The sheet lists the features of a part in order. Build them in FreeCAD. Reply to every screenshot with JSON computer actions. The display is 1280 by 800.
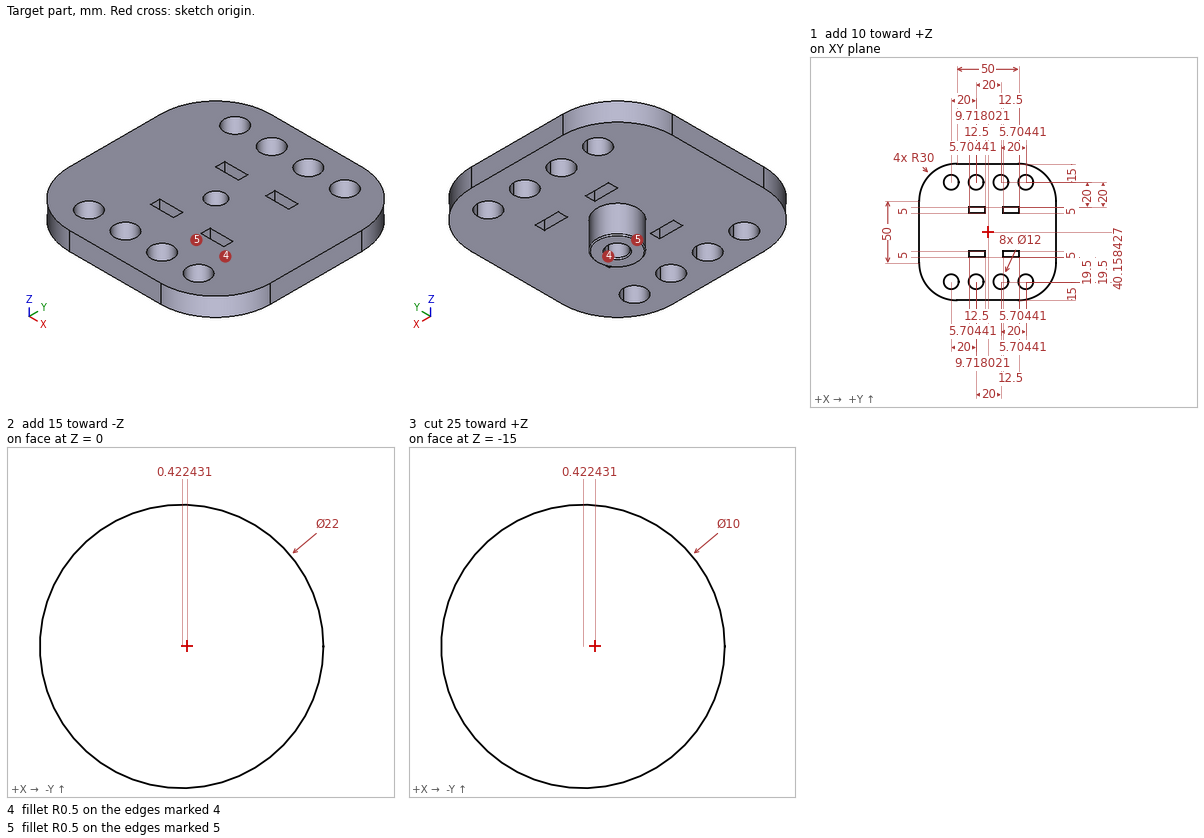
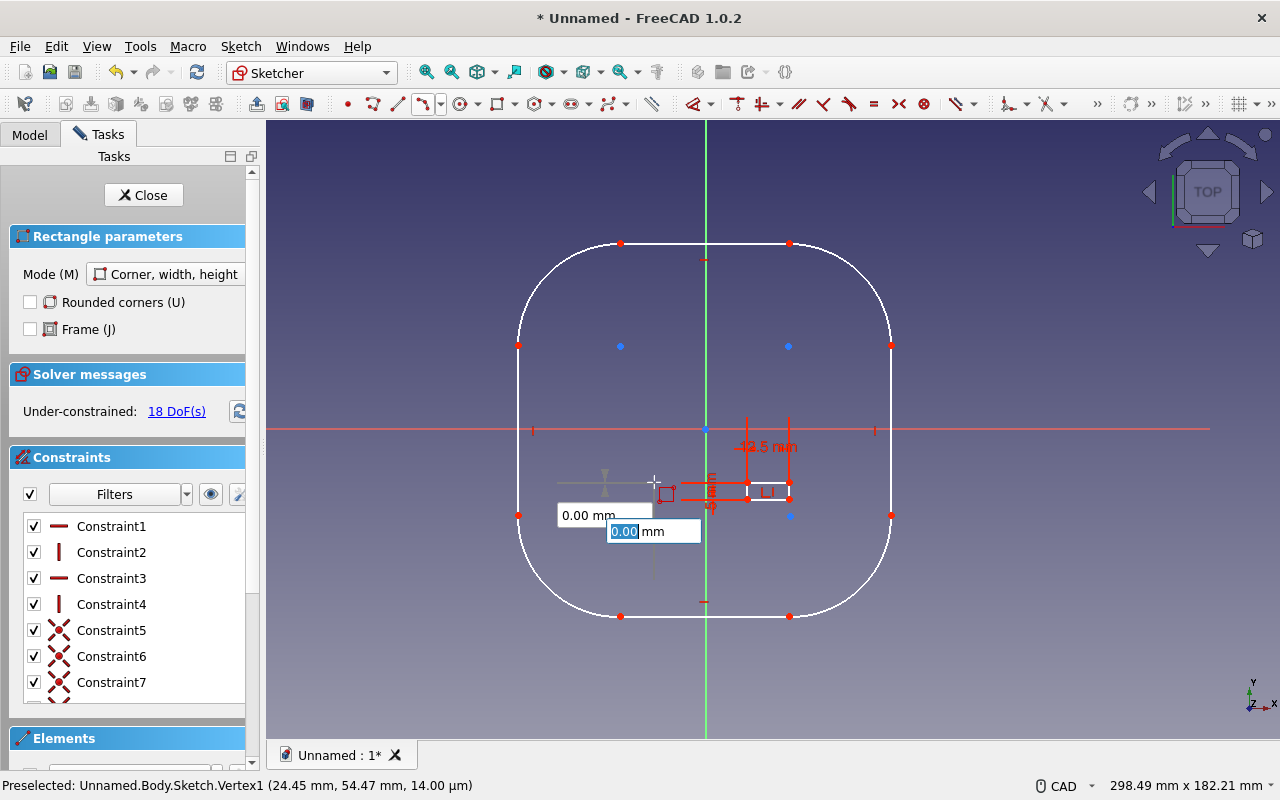
{"action": "scroll", "coordinate": [696, 499], "scroll_direction": "up", "scroll_amount": 3}
{"action": "mouse_move", "coordinate": [696, 499]}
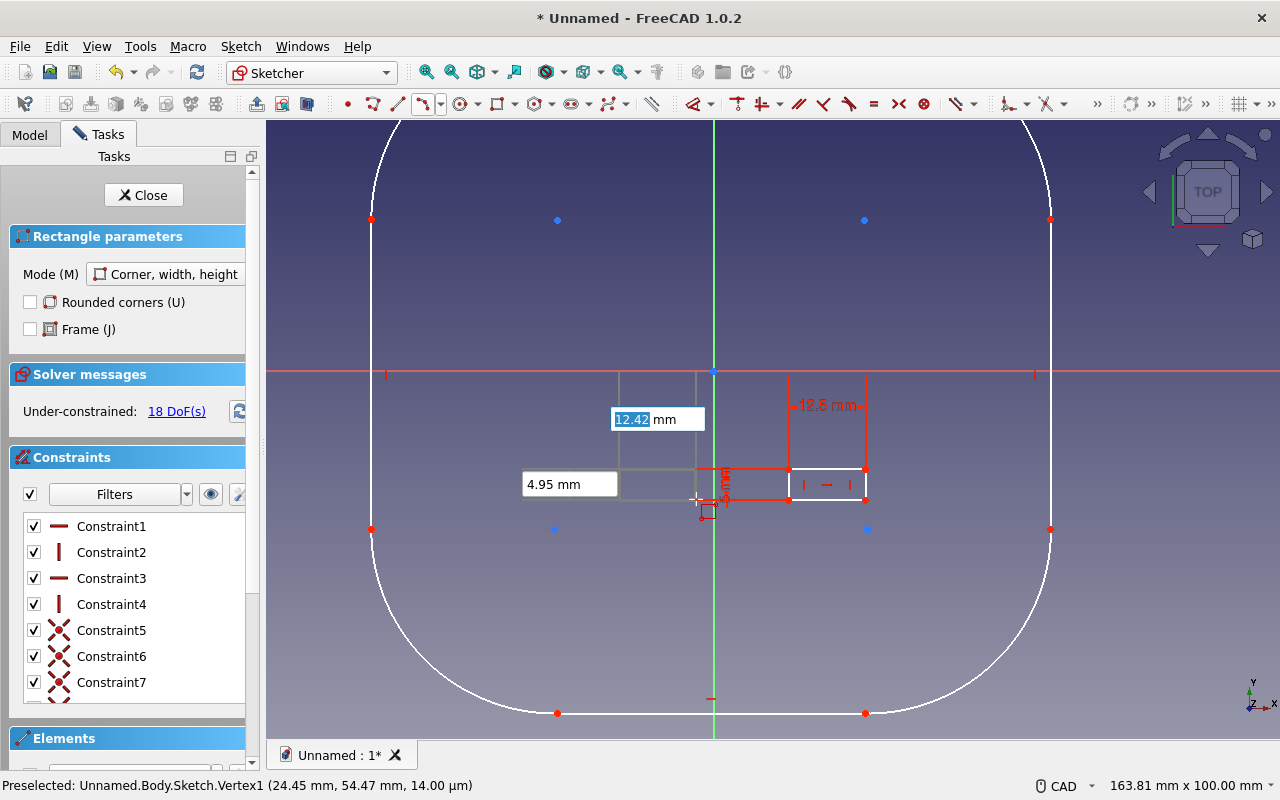
{"action": "type", "text": "12.5"}
{"action": "key", "text": "Tab"}
{"action": "type", "text": "5"}
{"action": "key", "text": "Return"}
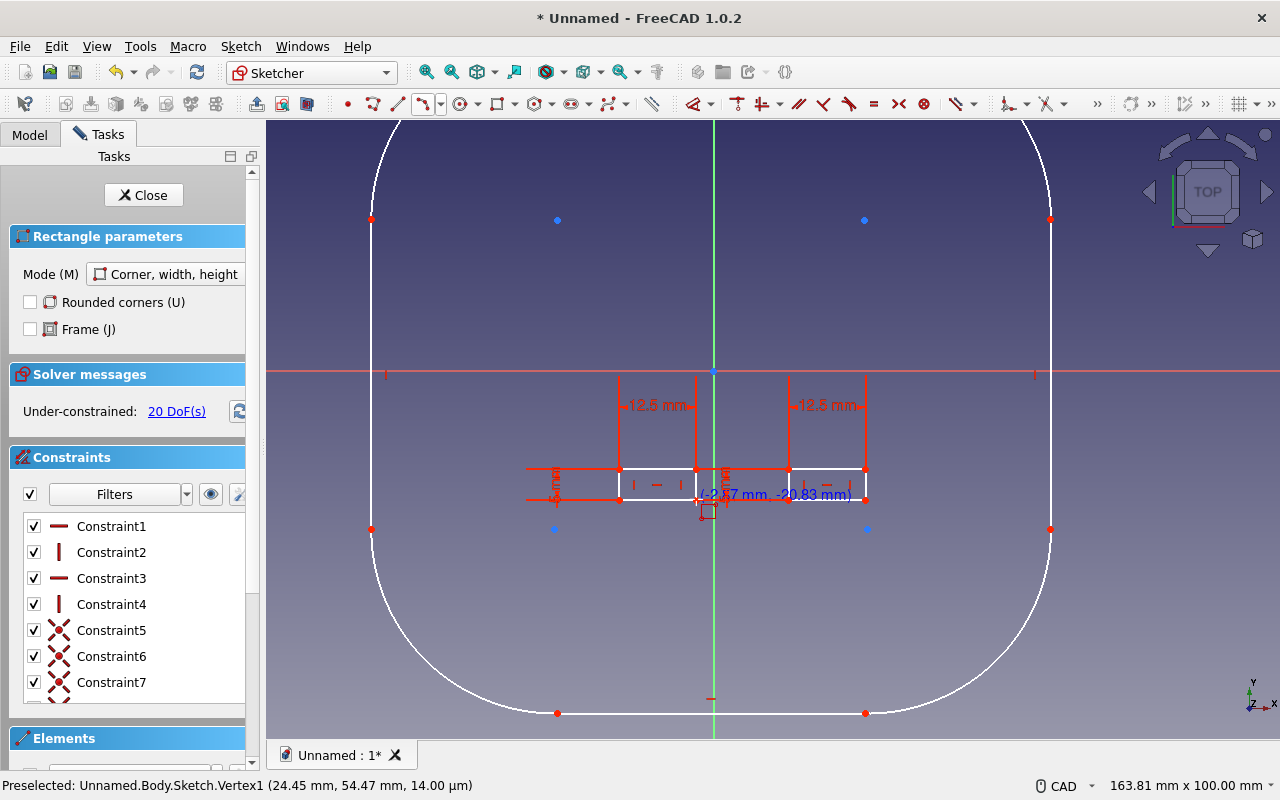
{"action": "left_click", "coordinate": [789, 248]}
{"action": "mouse_move", "coordinate": [866, 279]}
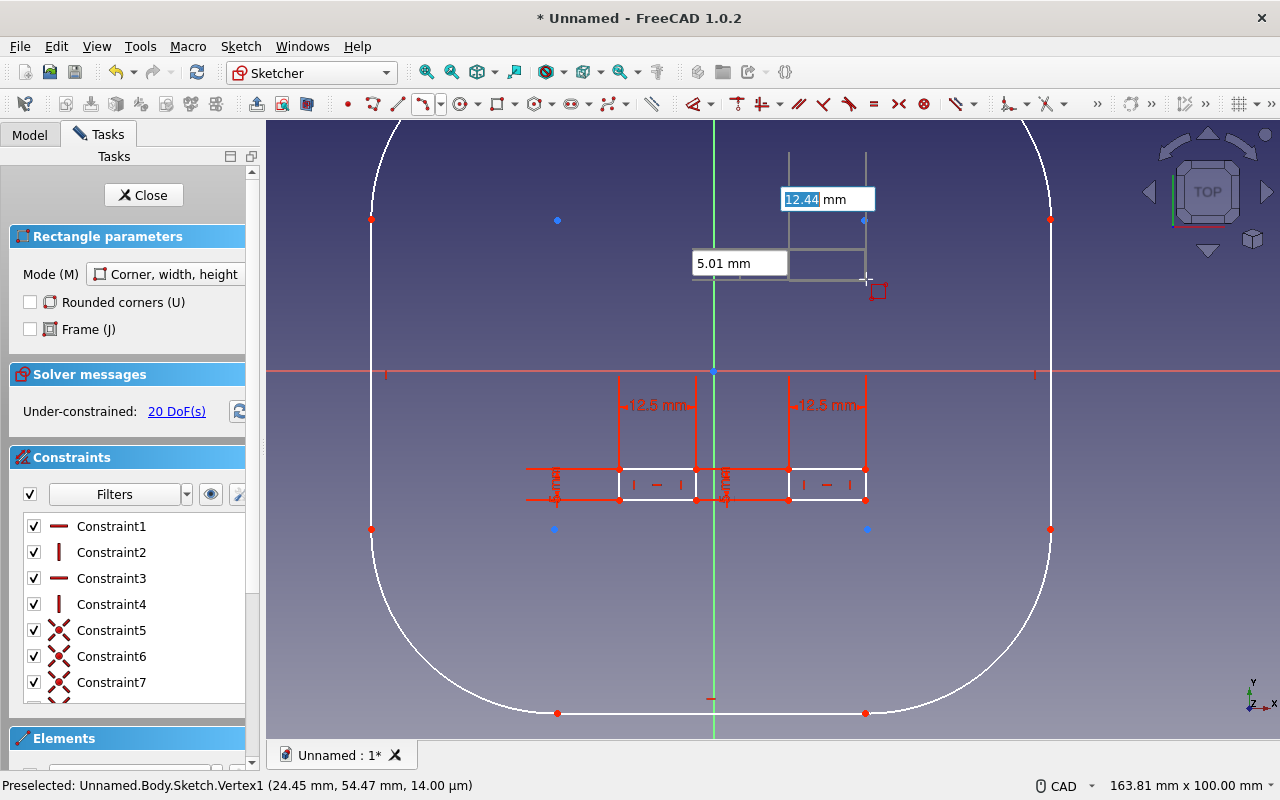
{"action": "type", "text": "12.5"}
{"action": "key", "text": "Tab"}
{"action": "type", "text": "5"}
{"action": "key", "text": "Return"}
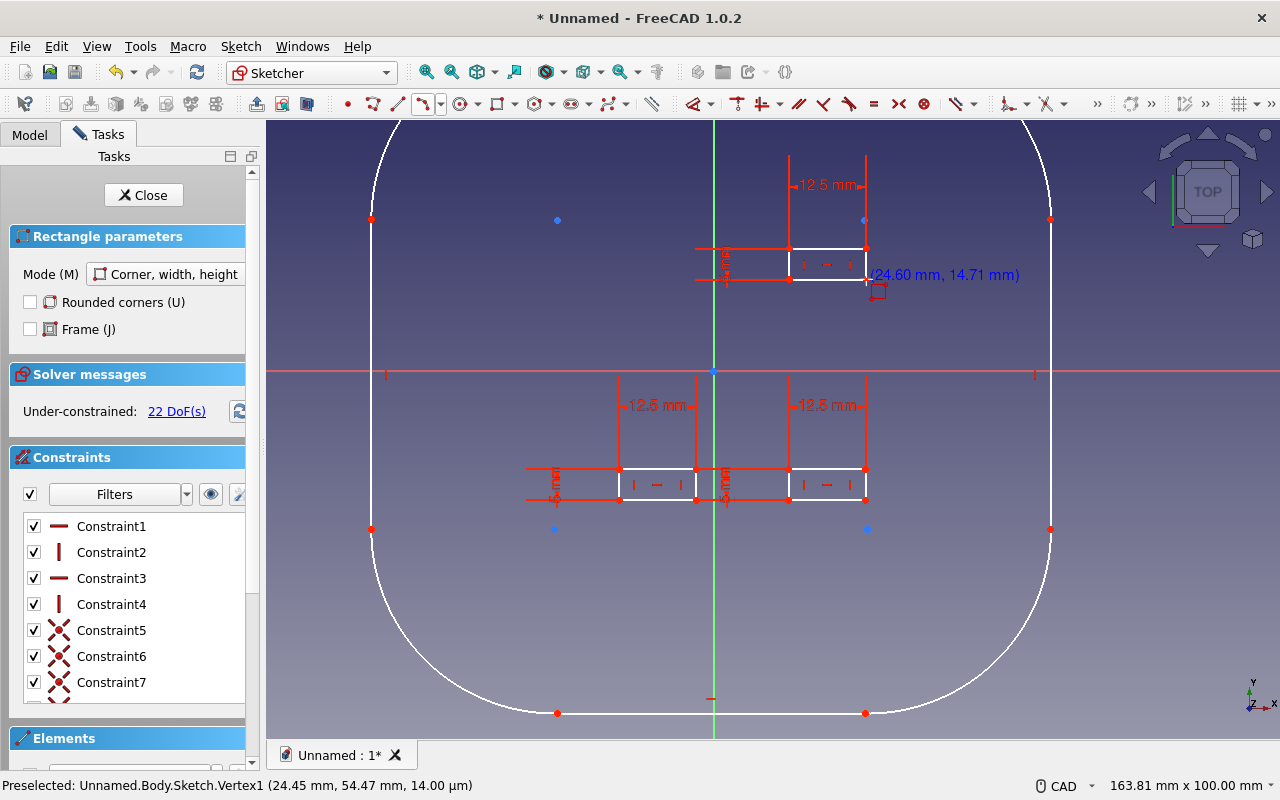
{"action": "left_click", "coordinate": [618, 248]}
{"action": "mouse_move", "coordinate": [696, 279]}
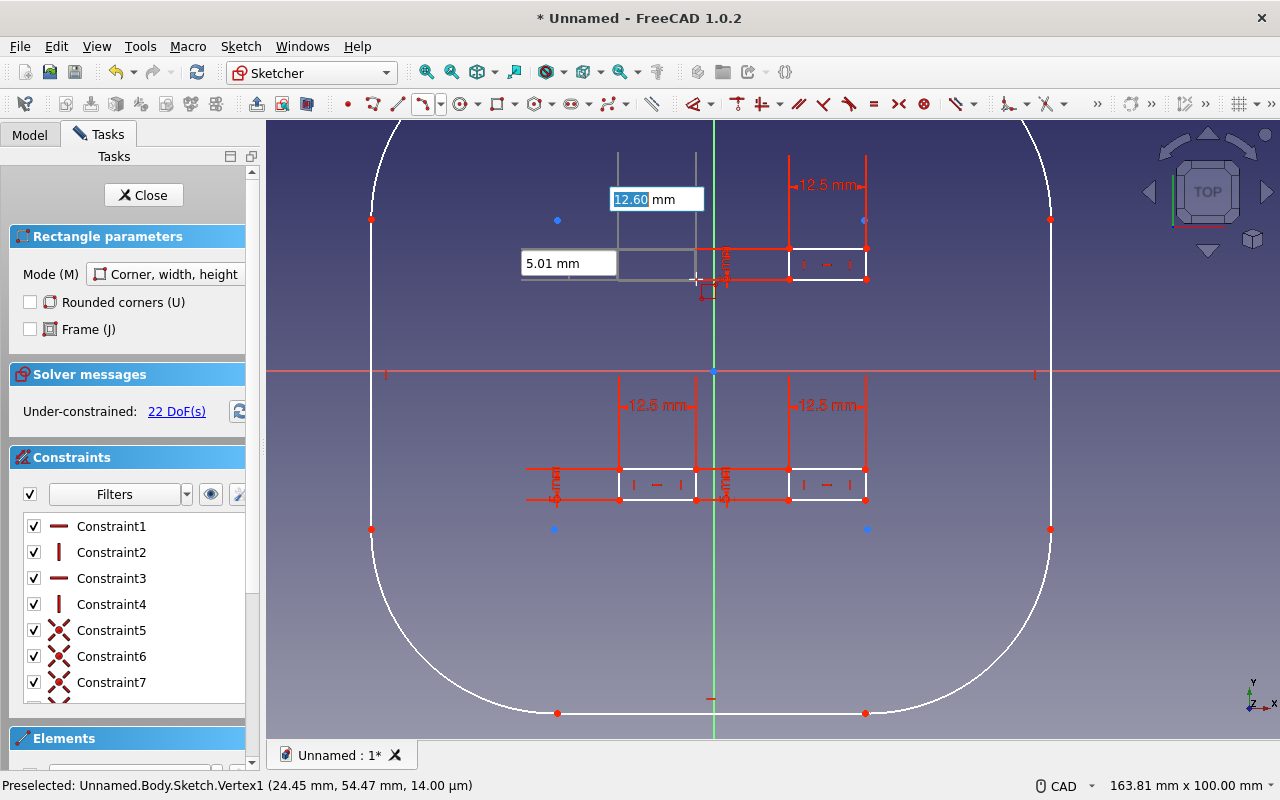
{"action": "type", "text": "12.5"}
{"action": "key", "text": "Tab"}
{"action": "type", "text": "5"}
{"action": "key", "text": "Return"}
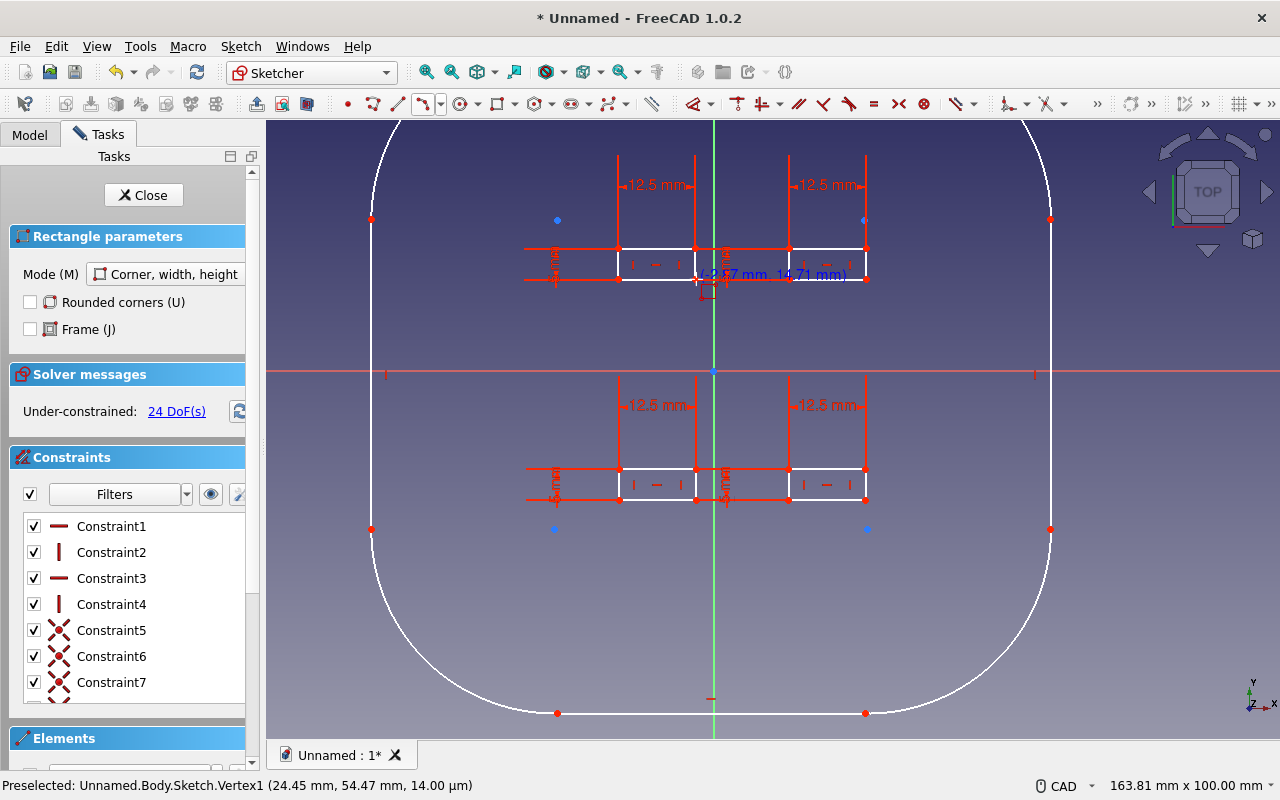
{"action": "key", "text": "g c"}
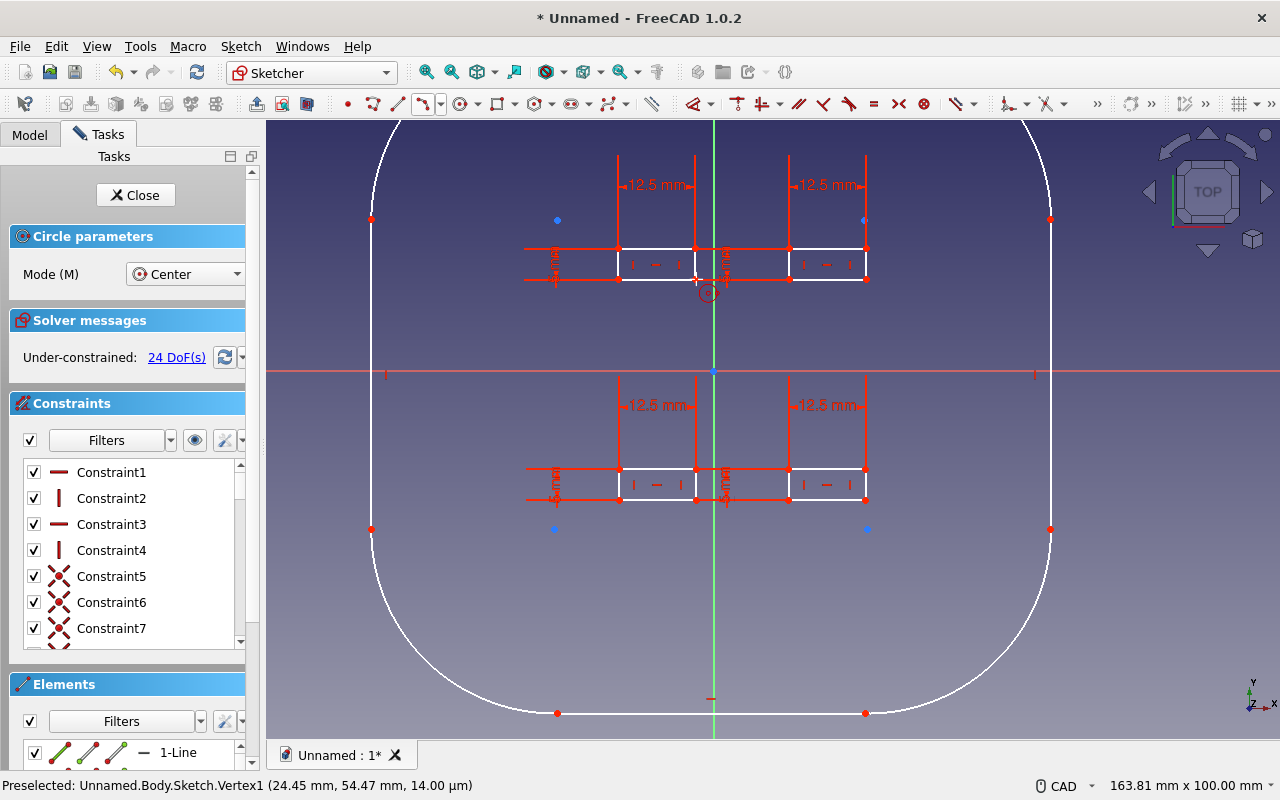
{"action": "left_click", "coordinate": [901, 620]}
{"action": "mouse_move", "coordinate": [927, 593]}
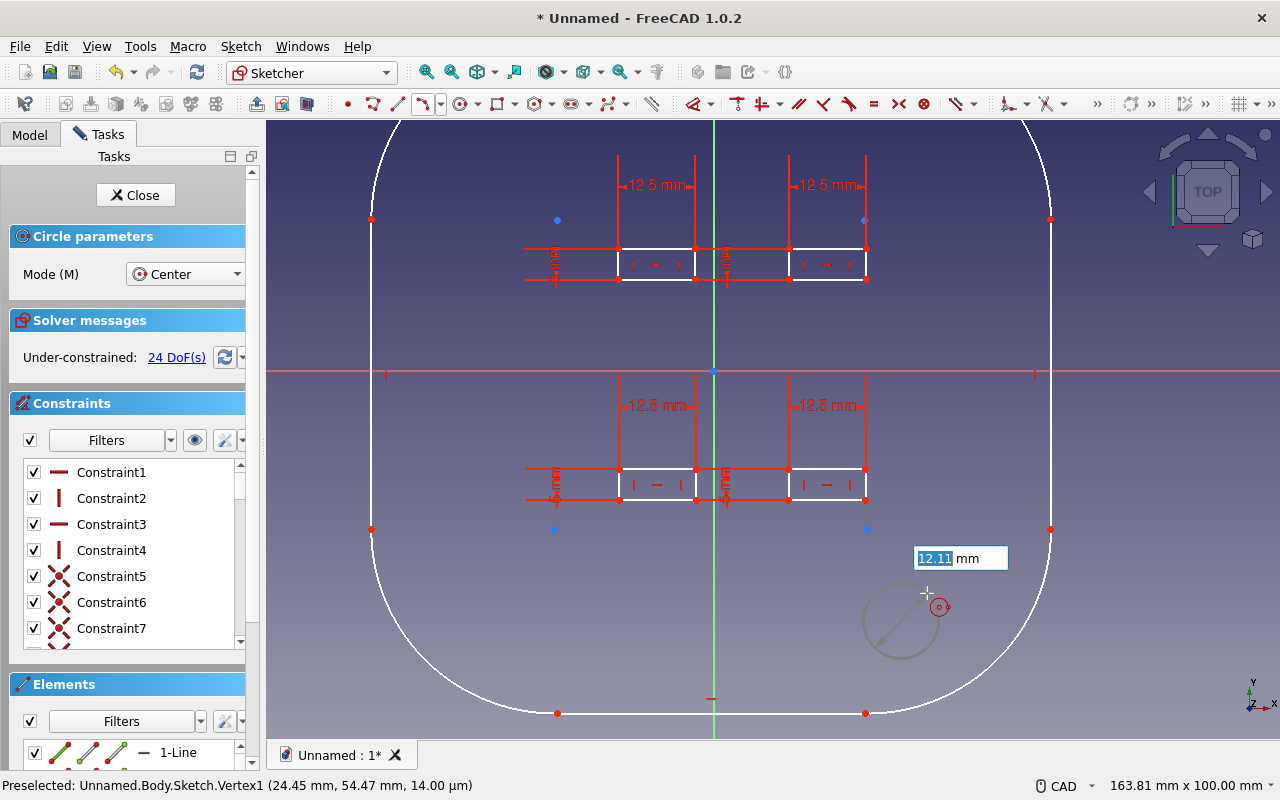
{"action": "type", "text": "12"}
{"action": "key", "text": "Return"}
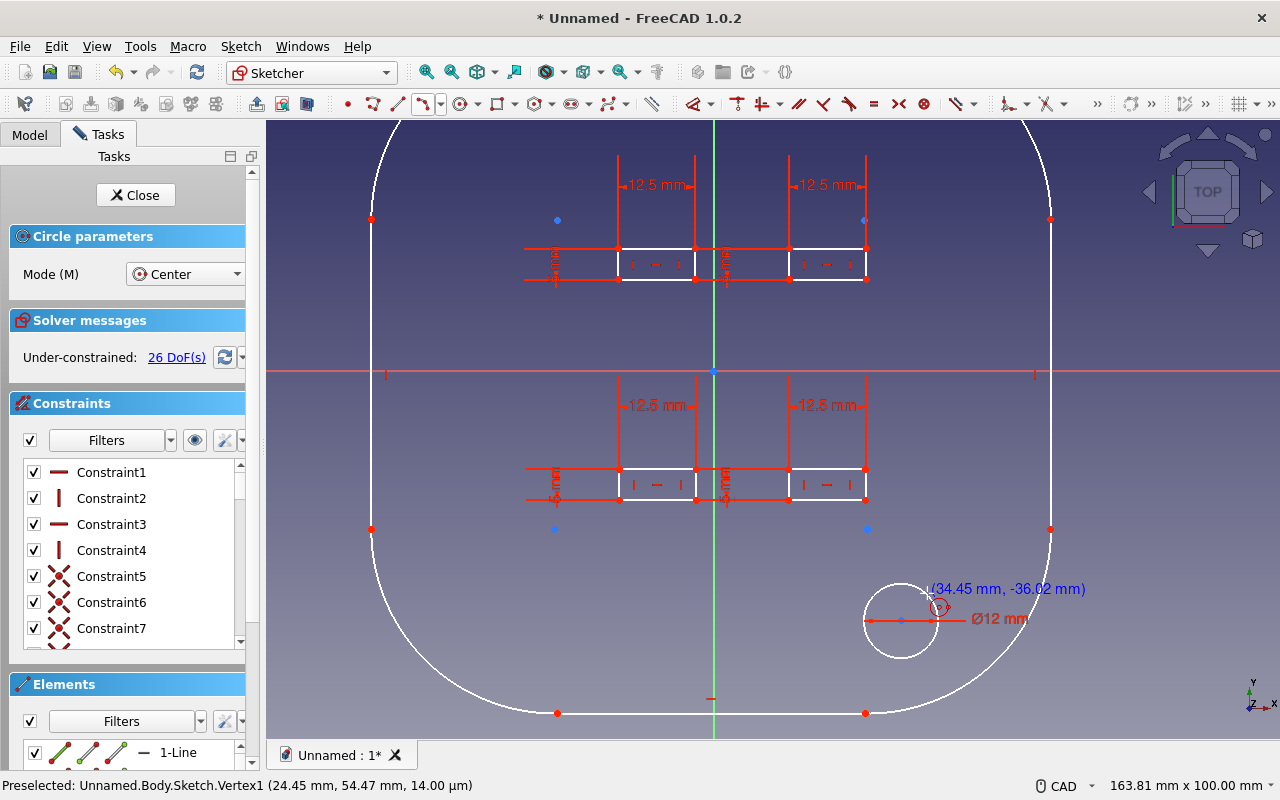
{"action": "left_click", "coordinate": [777, 620]}
{"action": "mouse_move", "coordinate": [804, 593]}